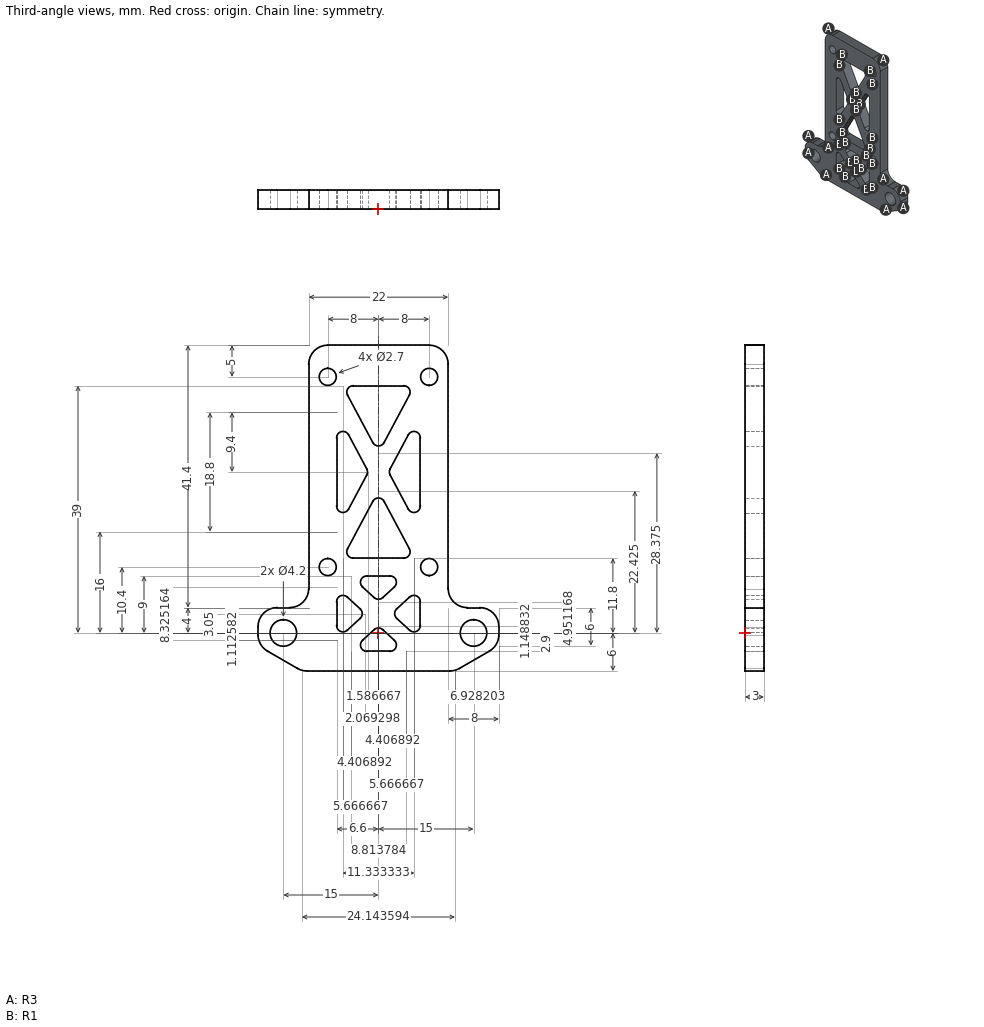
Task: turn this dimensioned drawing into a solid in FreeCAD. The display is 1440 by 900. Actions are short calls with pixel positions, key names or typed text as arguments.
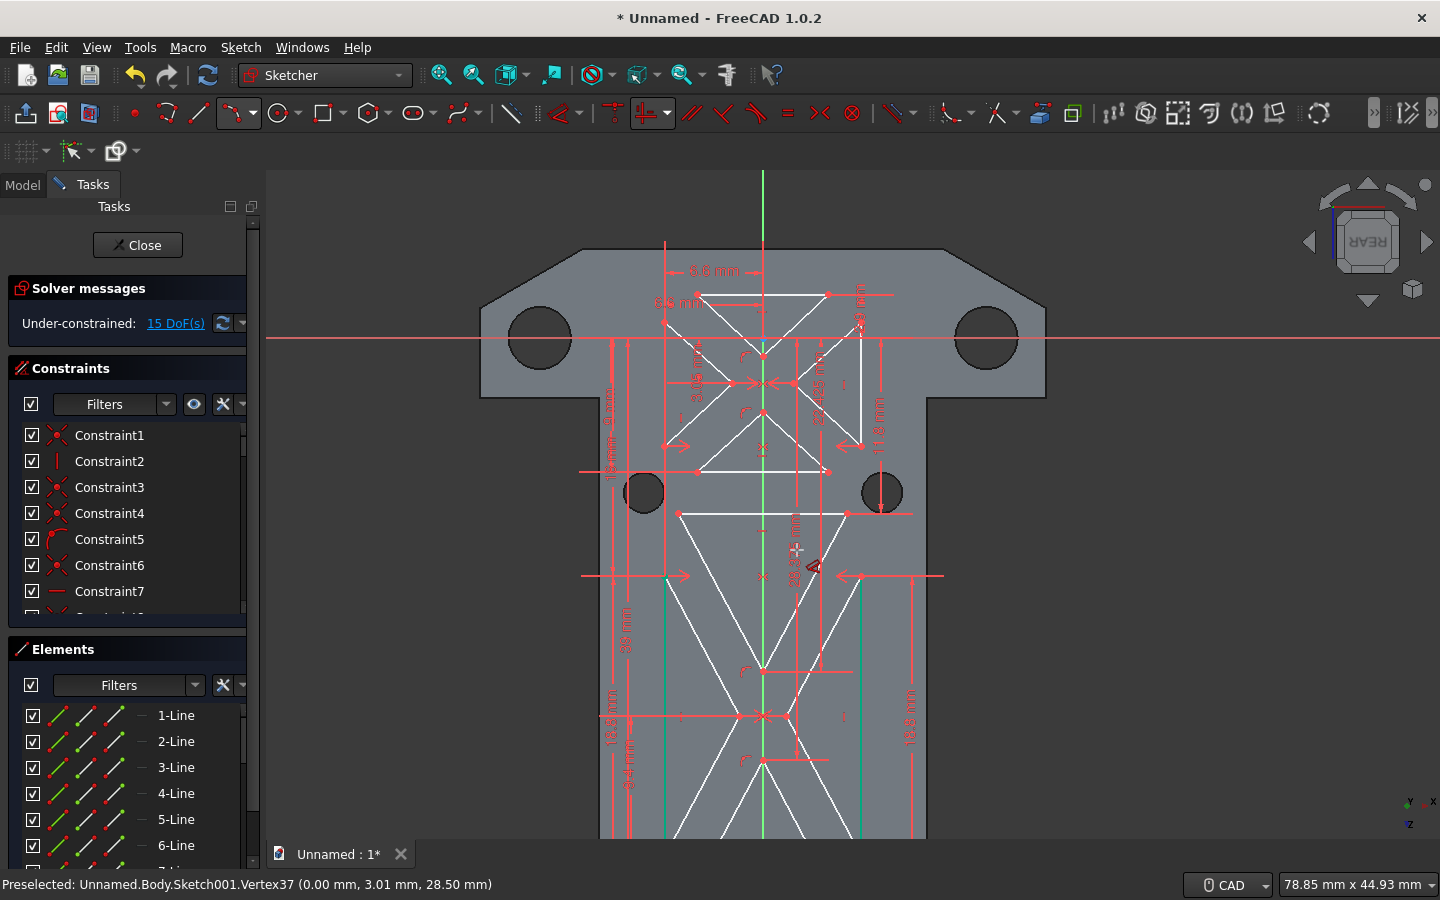
click(665, 360)
click(631, 428)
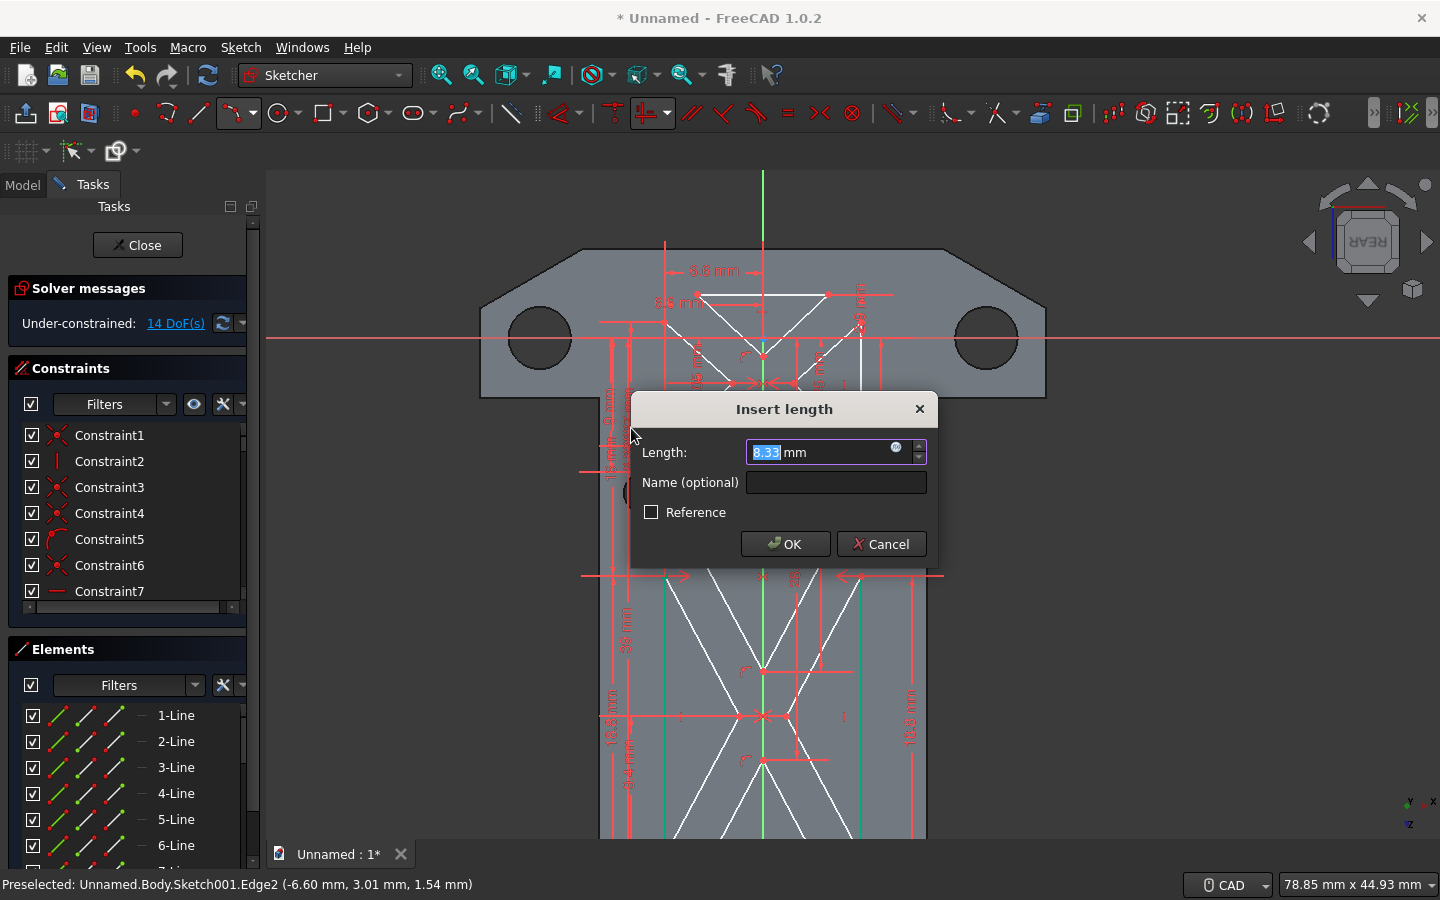
text(8.325164)
key(Return)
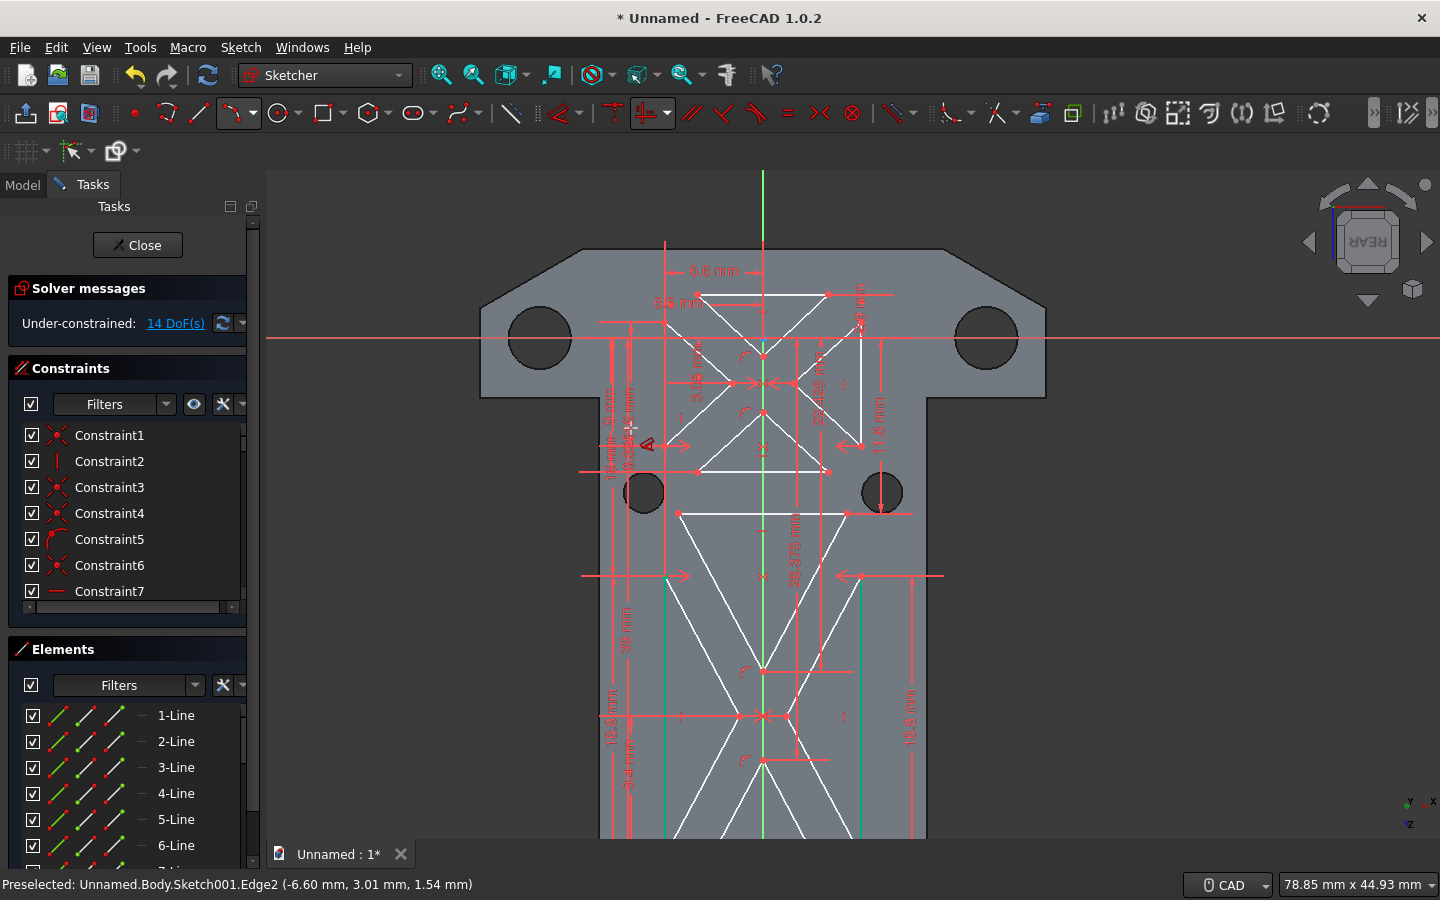
click(789, 295)
click(793, 261)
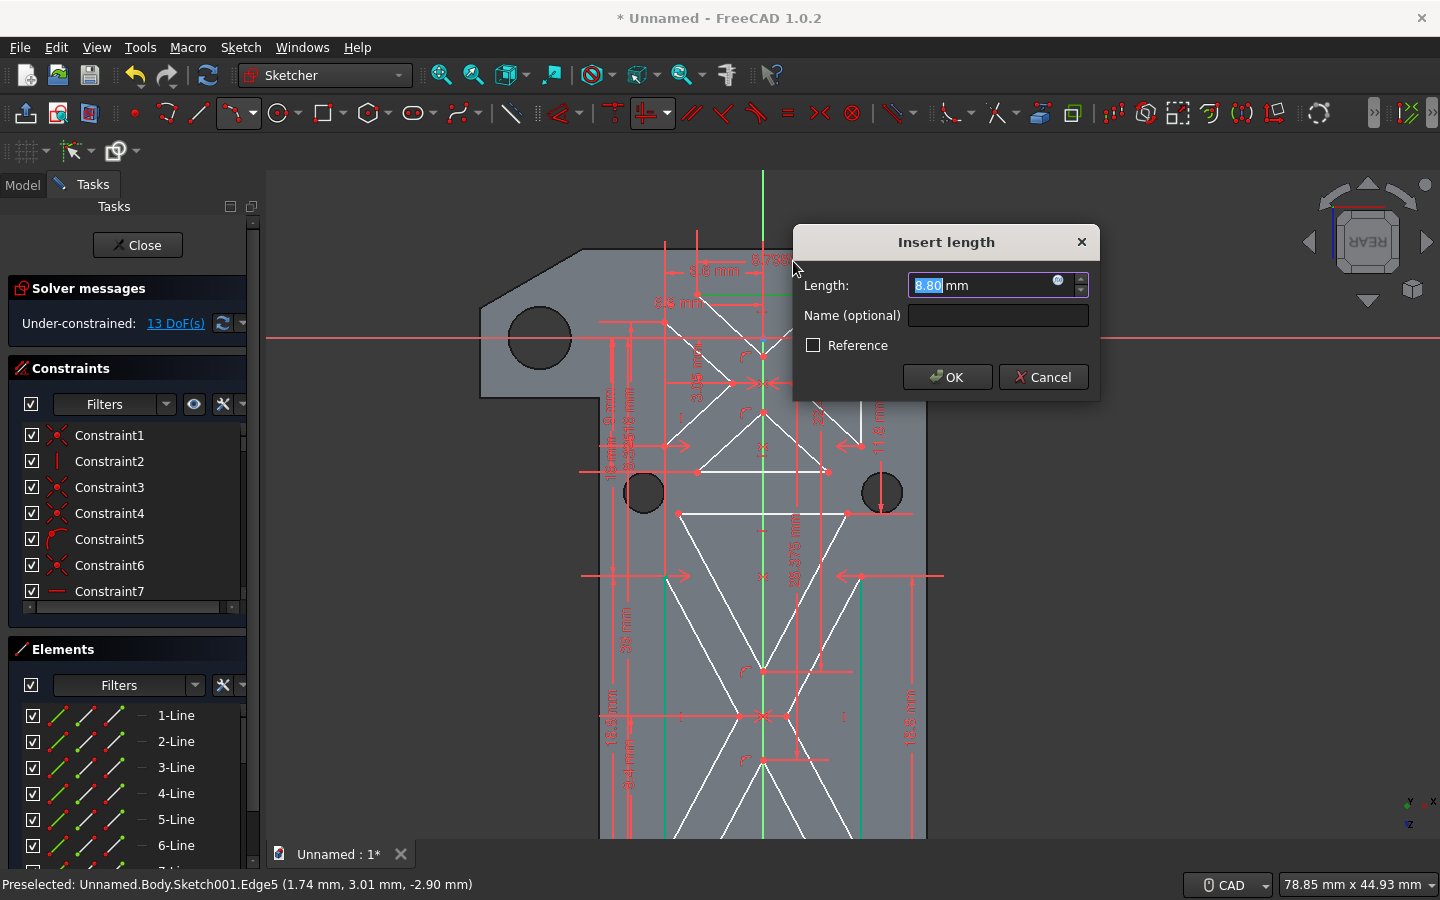
text(8.813784)
key(Return)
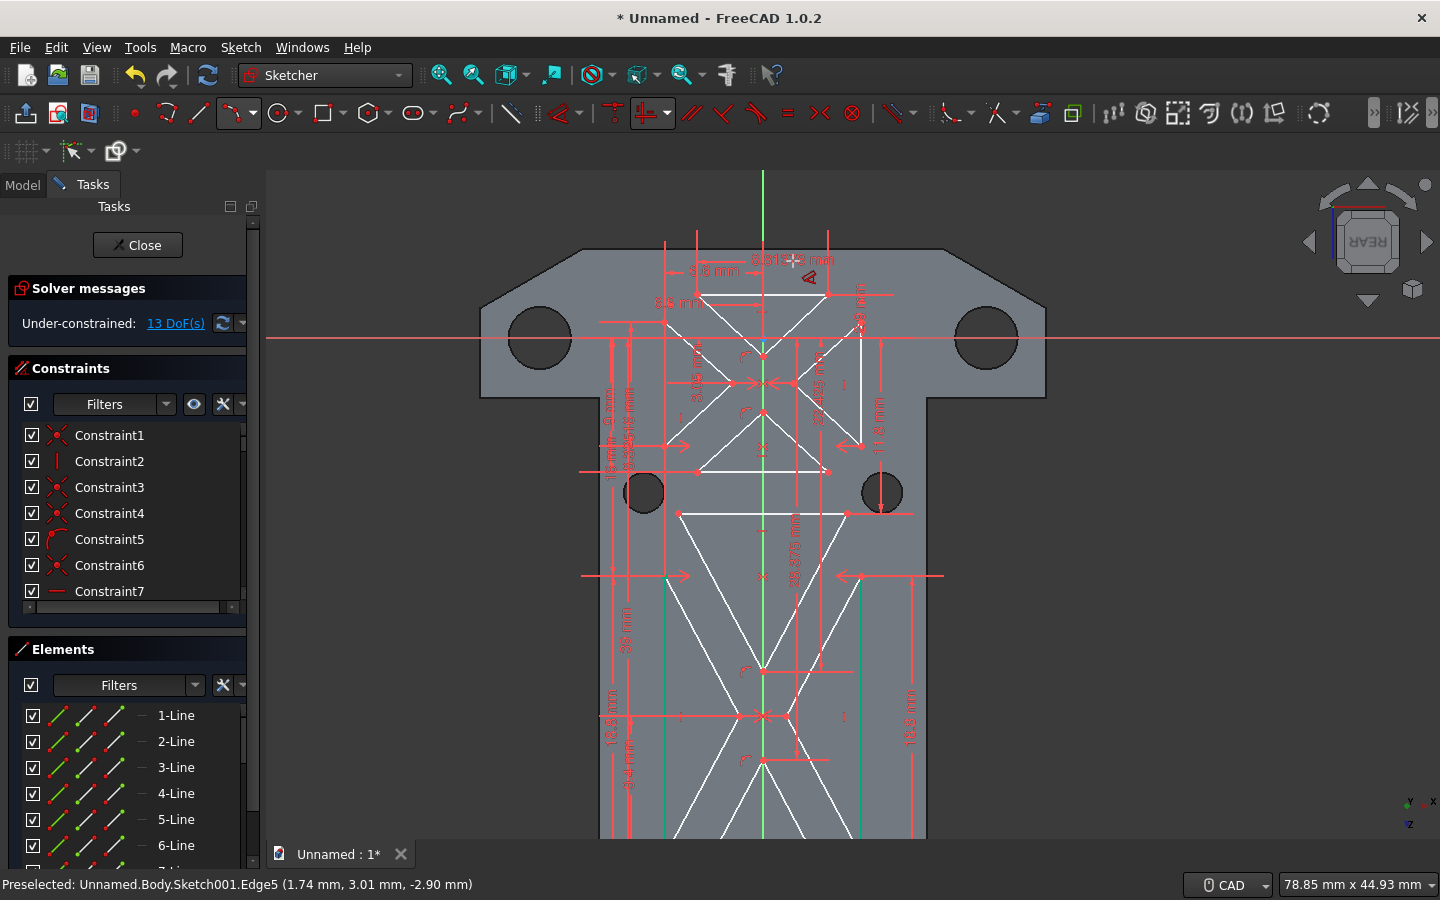
click(861, 409)
click(895, 384)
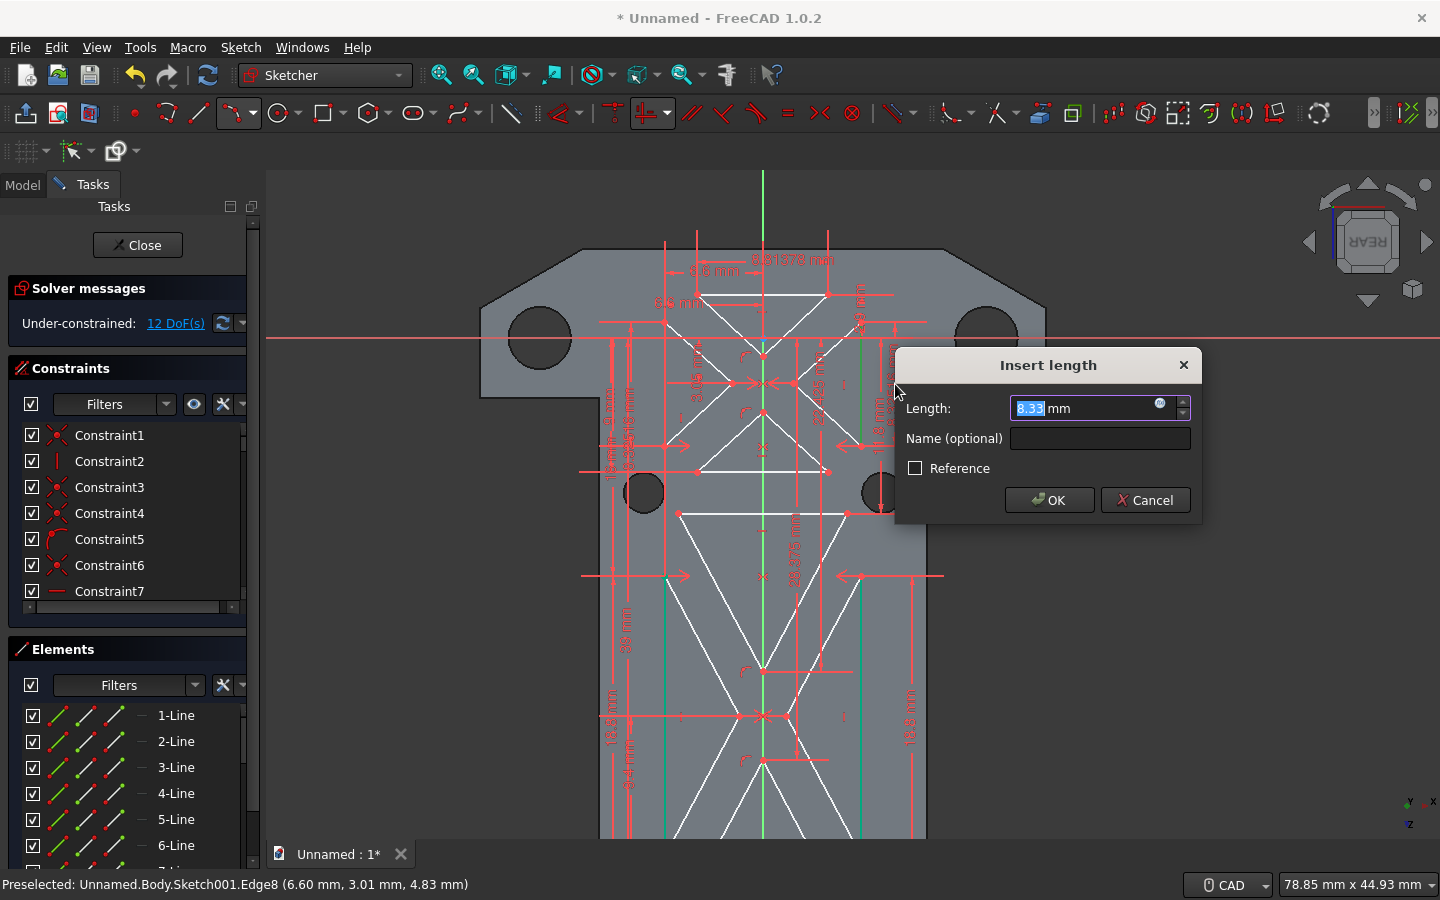
text(8.325164)
key(Return)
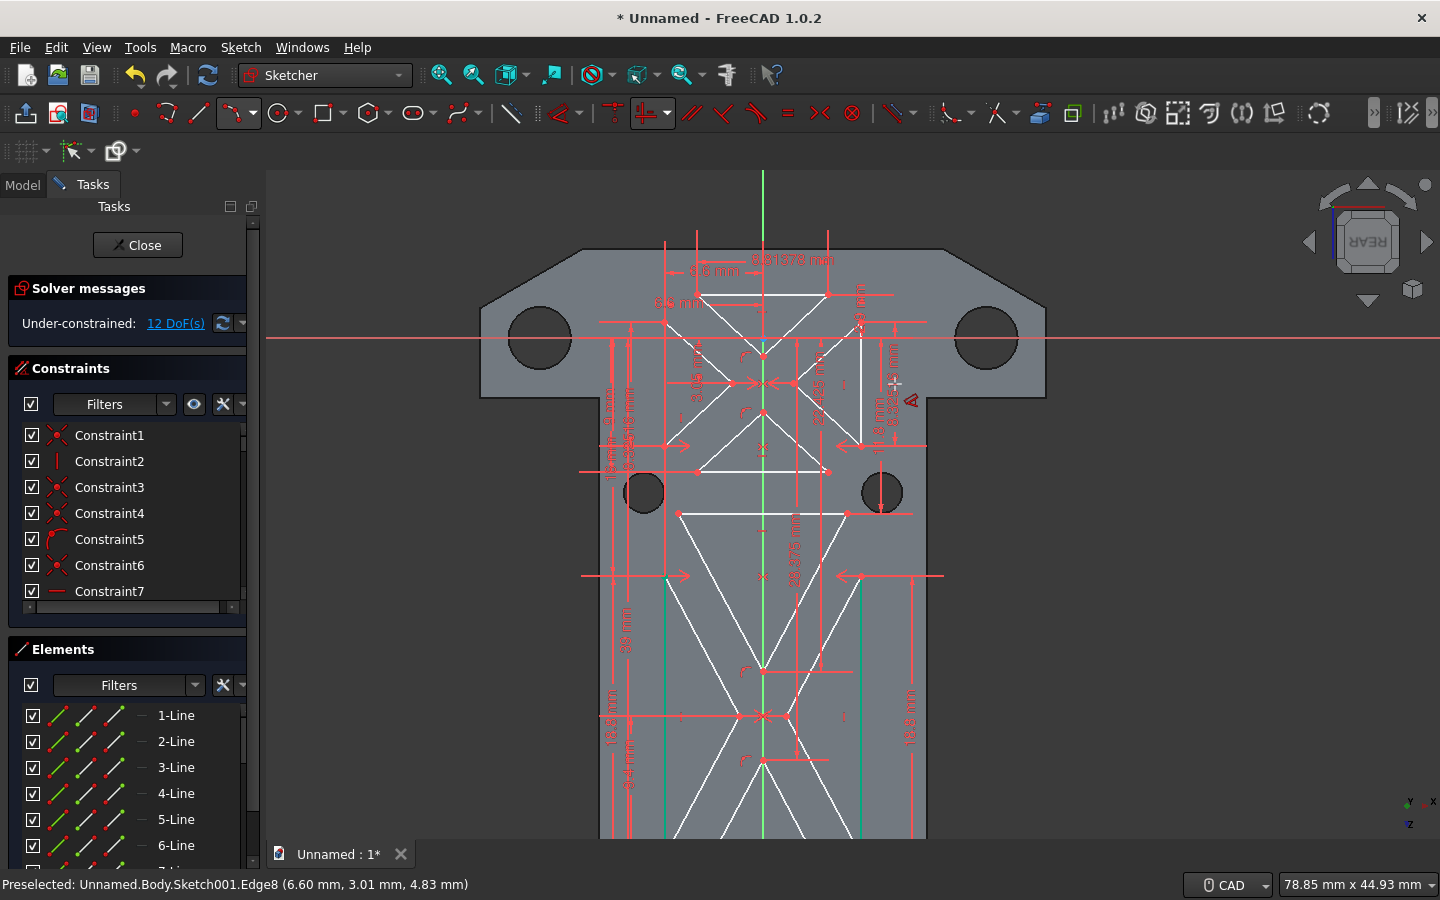
click(737, 472)
click(733, 414)